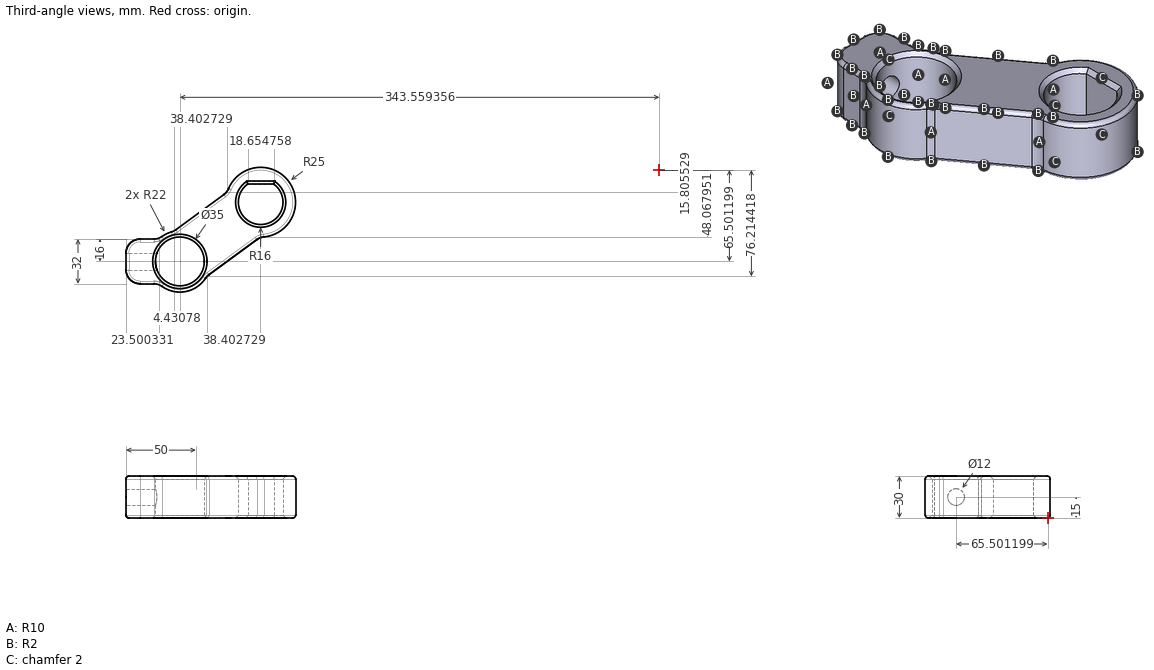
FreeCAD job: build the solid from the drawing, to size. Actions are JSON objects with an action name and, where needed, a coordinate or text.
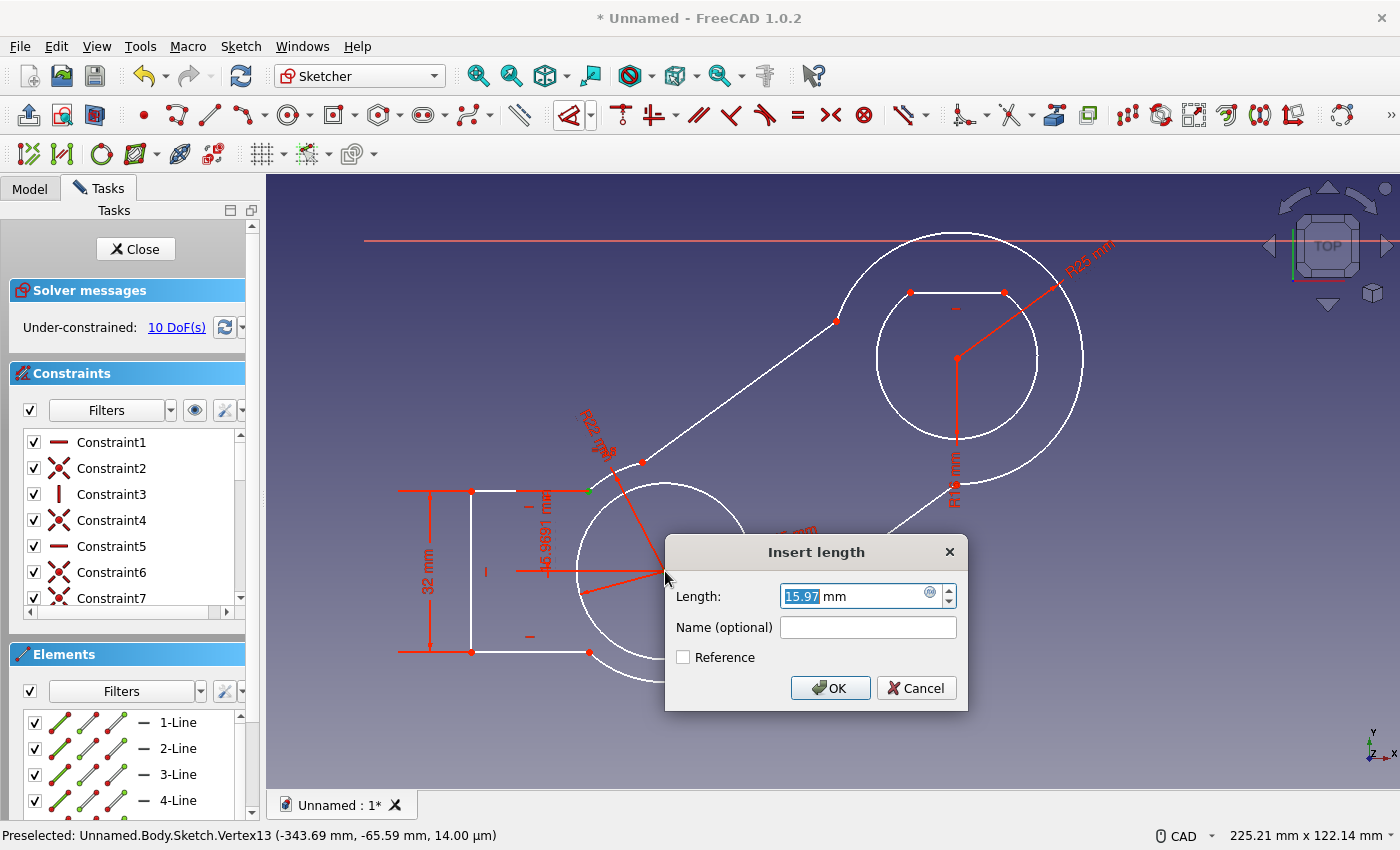
{"action": "type", "text": "16"}
{"action": "key", "text": "Return"}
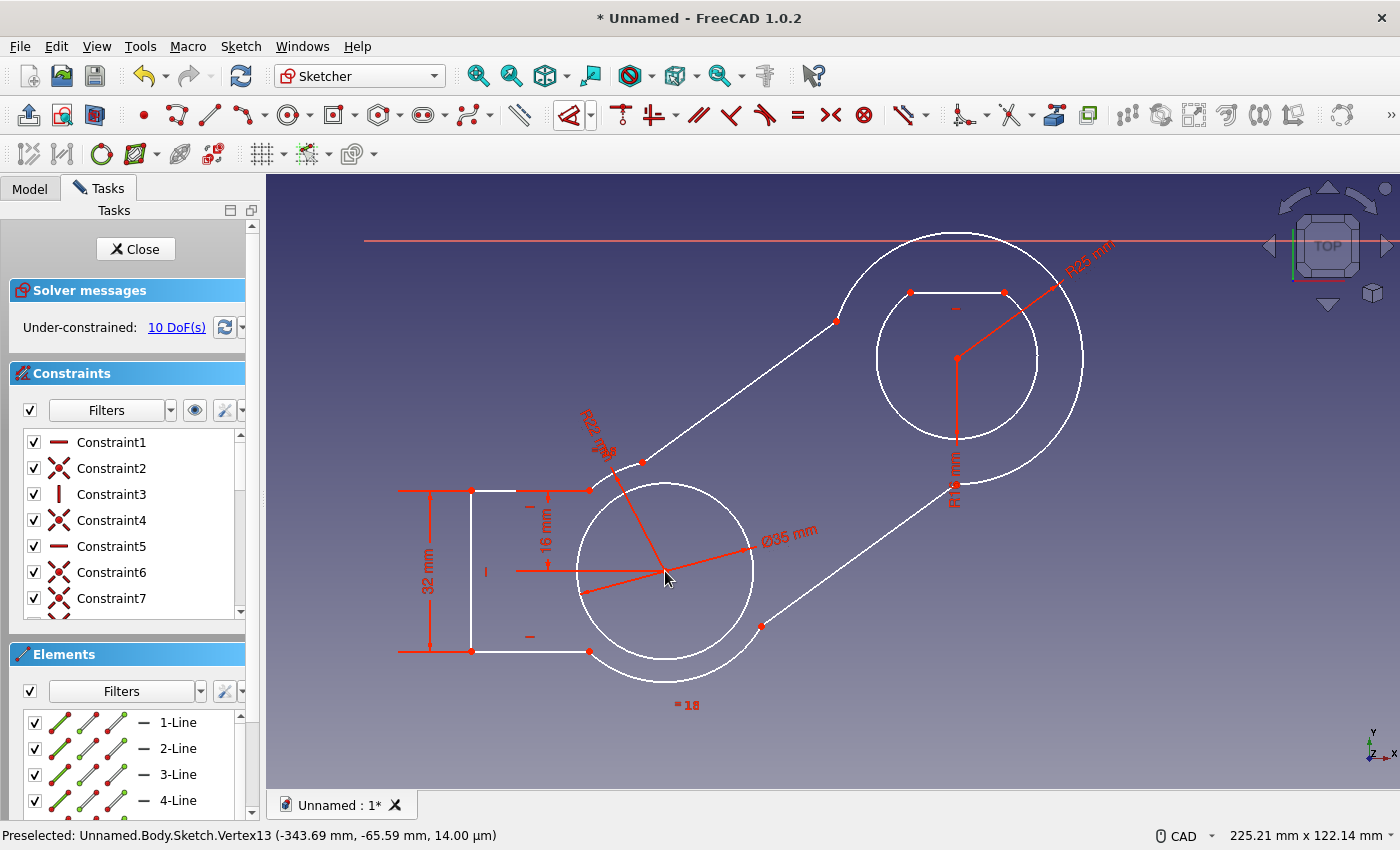
{"action": "scroll", "coordinate": [643, 463], "scroll_direction": "up", "scroll_amount": 3}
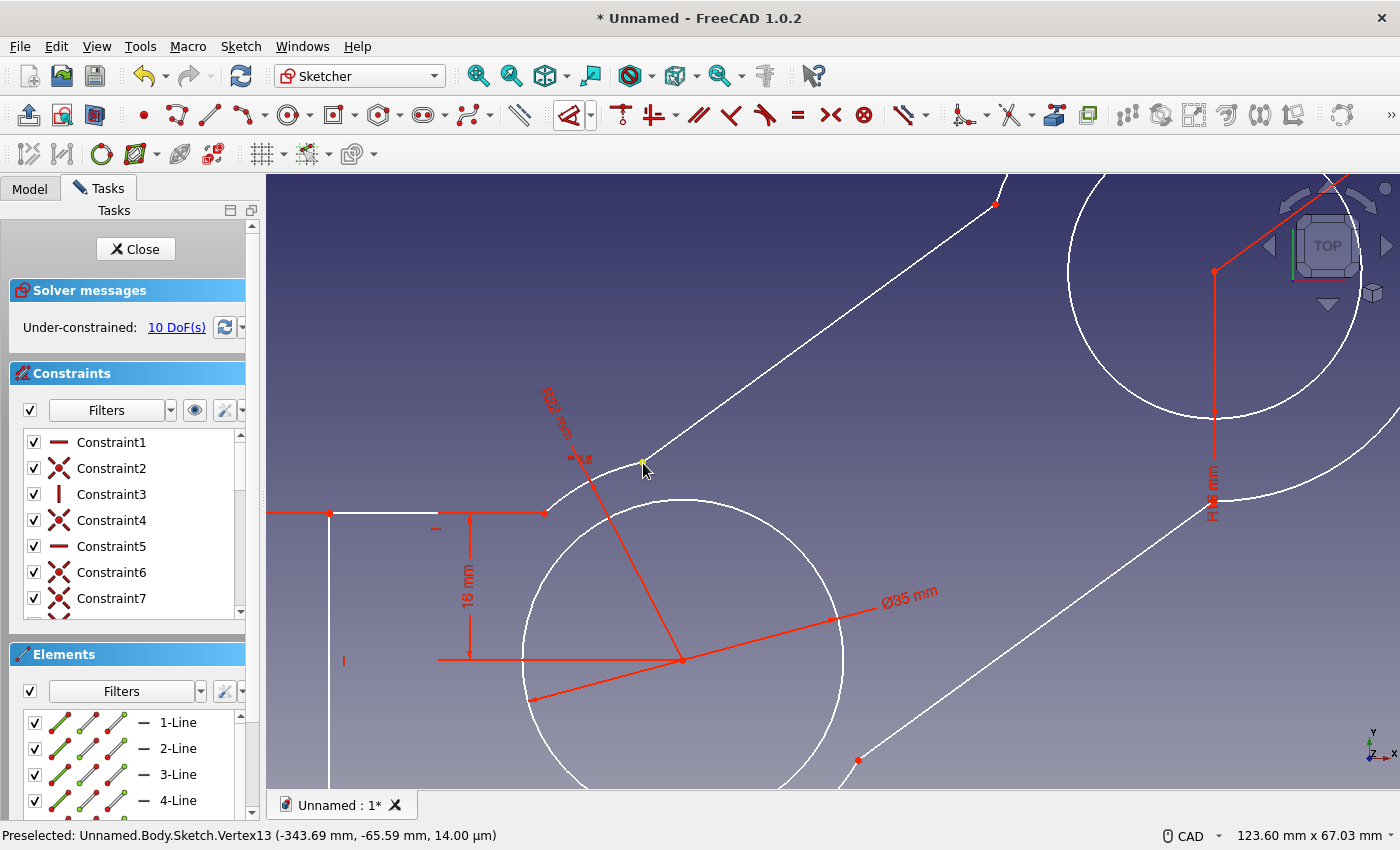
{"action": "left_click", "coordinate": [643, 462]}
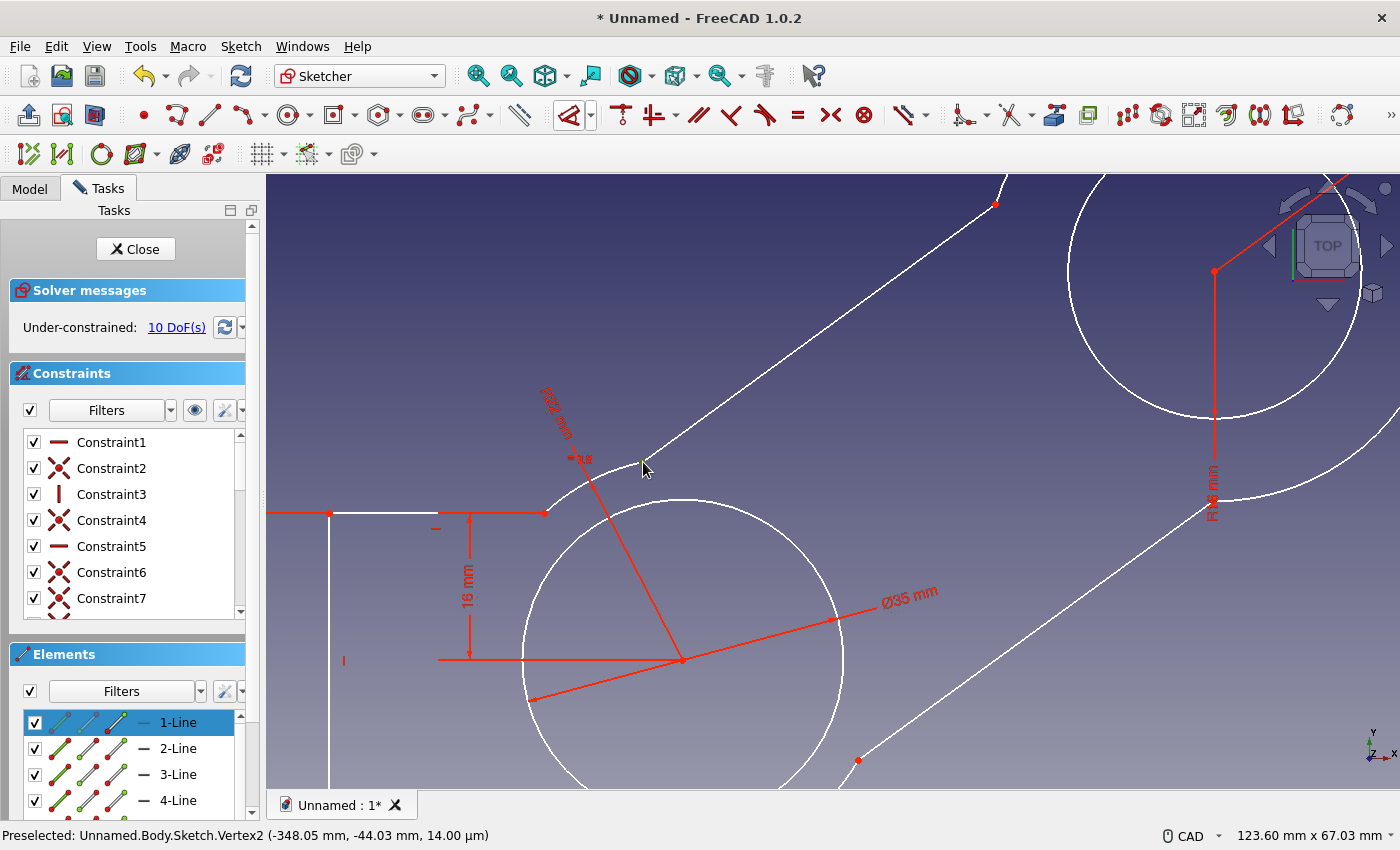
{"action": "left_click", "coordinate": [683, 660]}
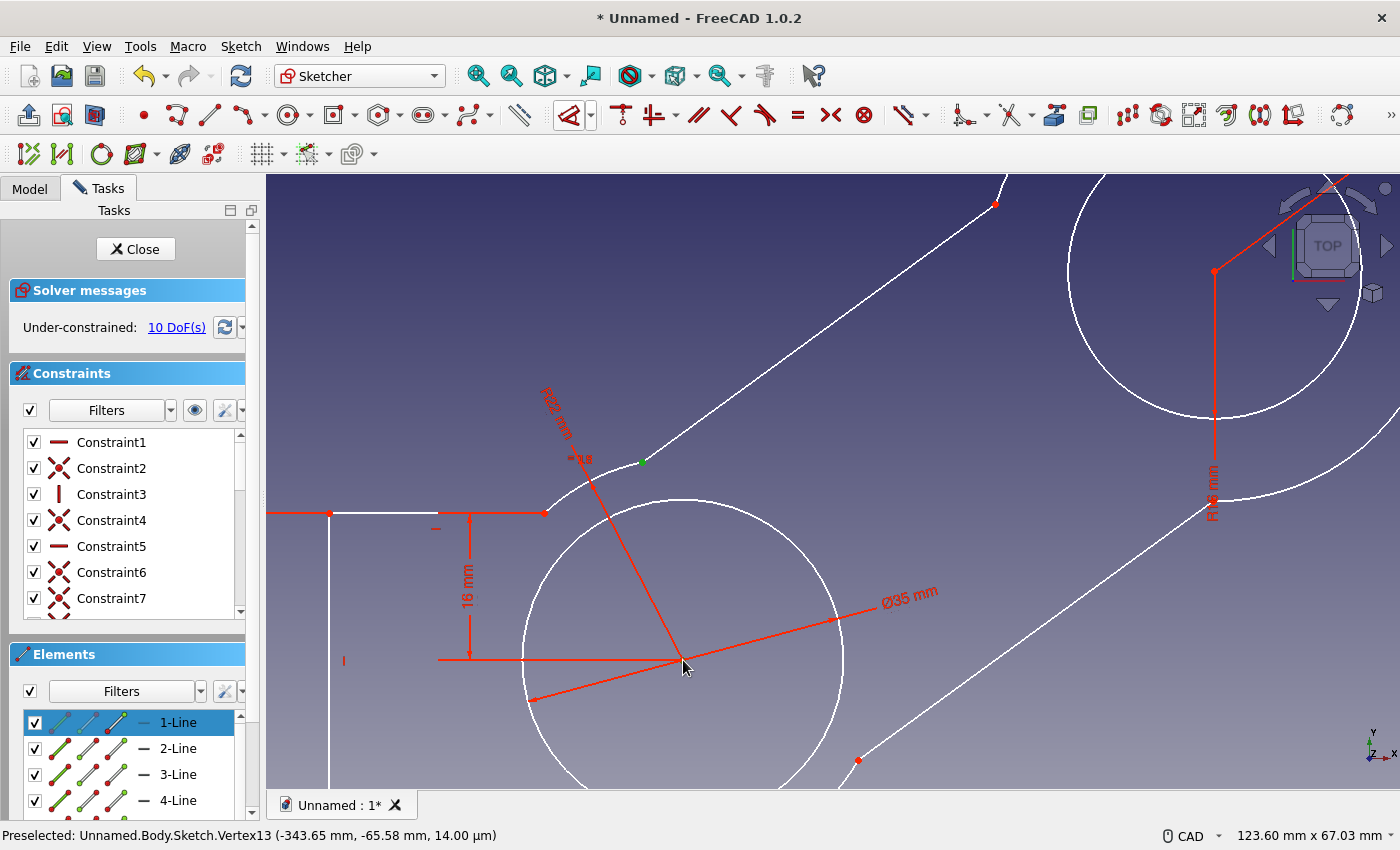
{"action": "left_click", "coordinate": [590, 116]}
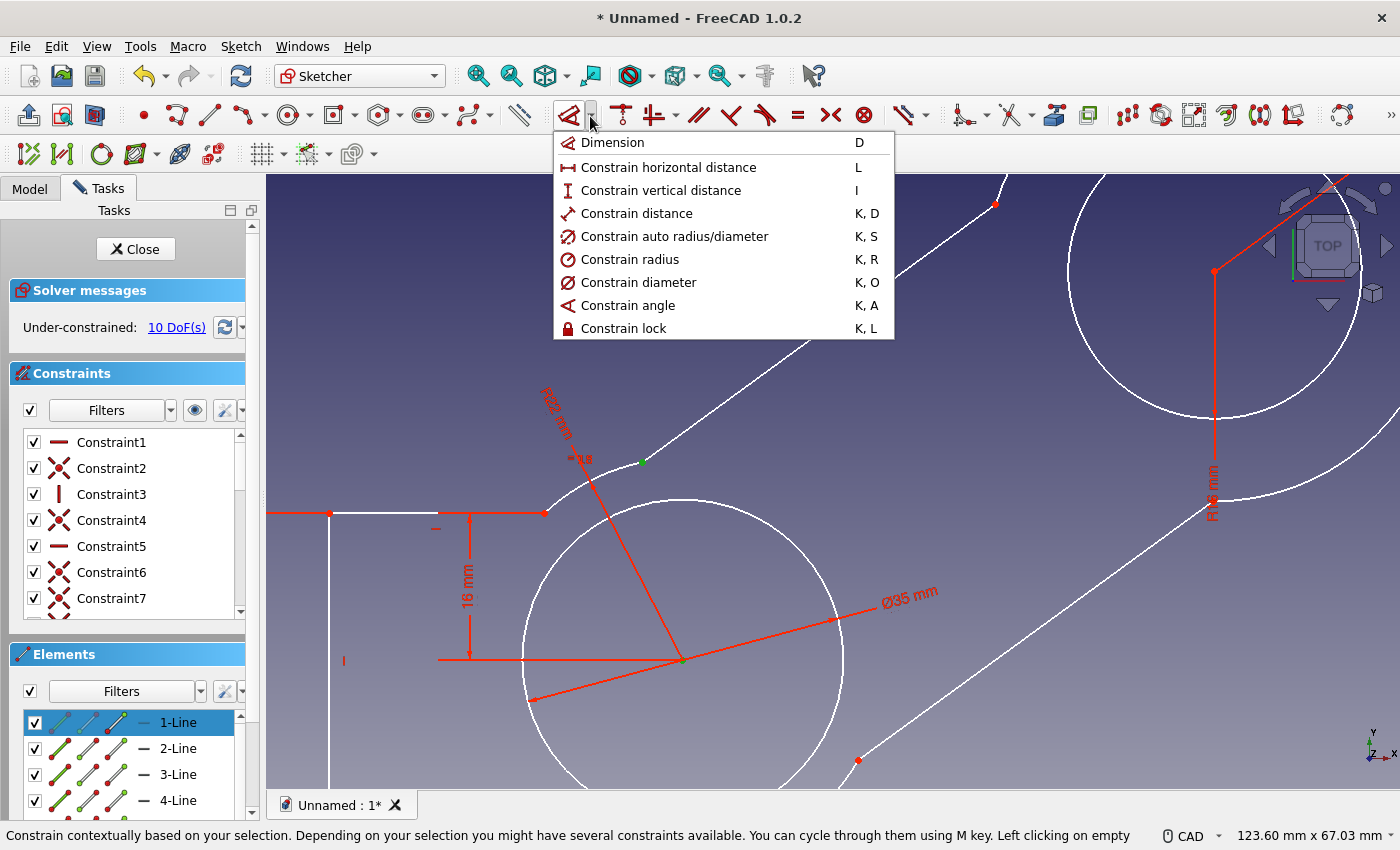
{"action": "left_click", "coordinate": [724, 168]}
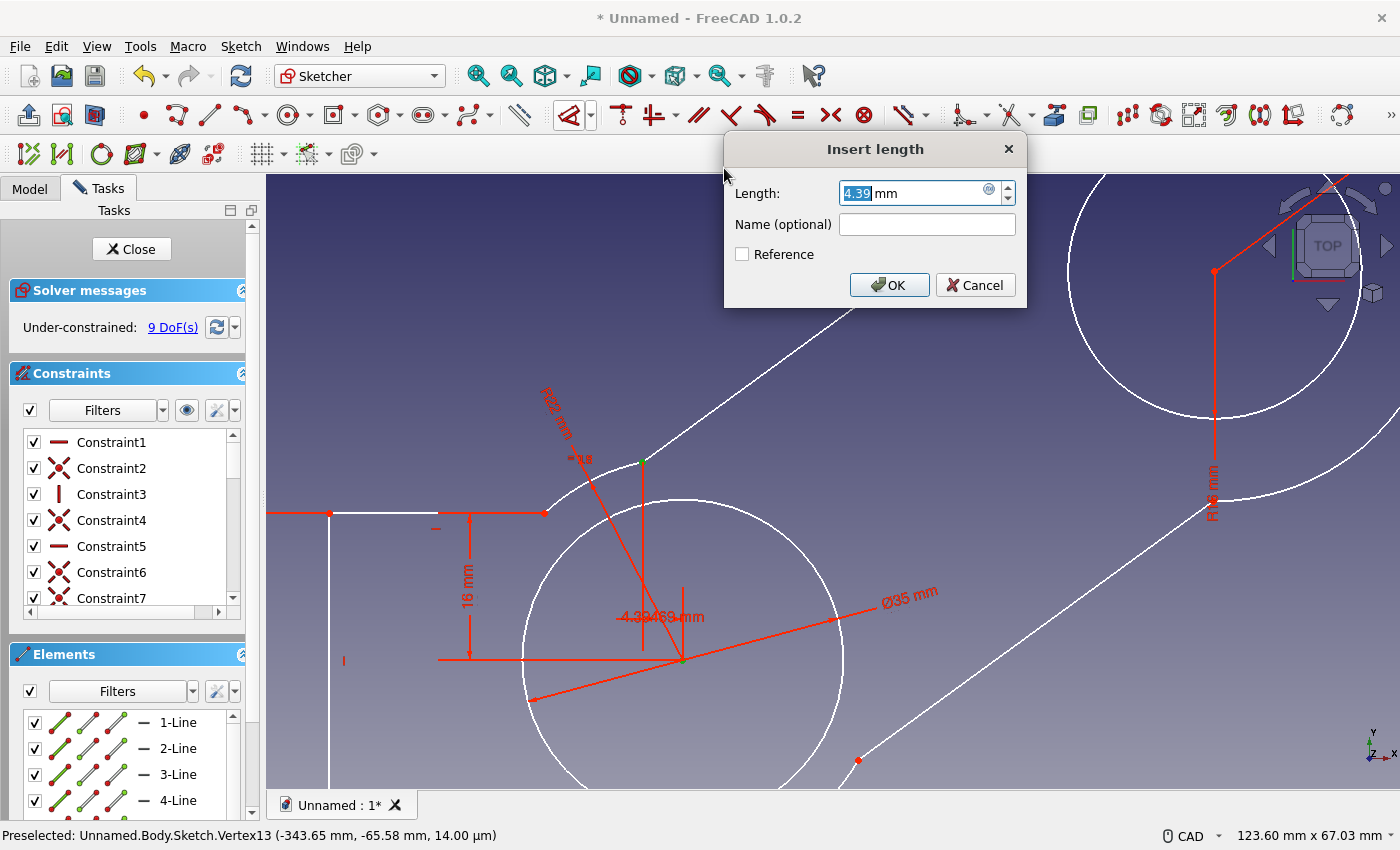
{"action": "type", "text": "4.43078"}
{"action": "key", "text": "Return"}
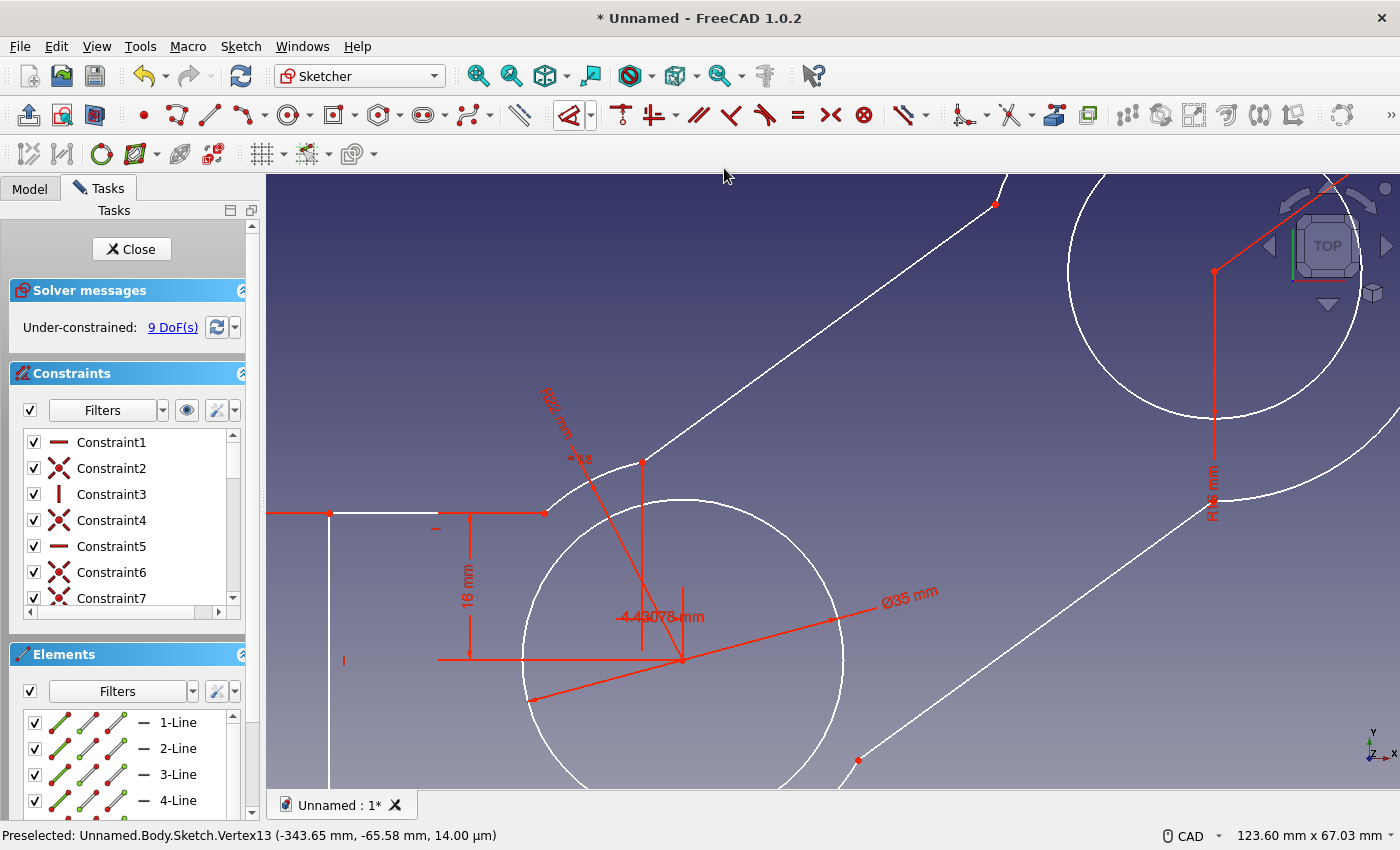
{"action": "left_click", "coordinate": [480, 513]}